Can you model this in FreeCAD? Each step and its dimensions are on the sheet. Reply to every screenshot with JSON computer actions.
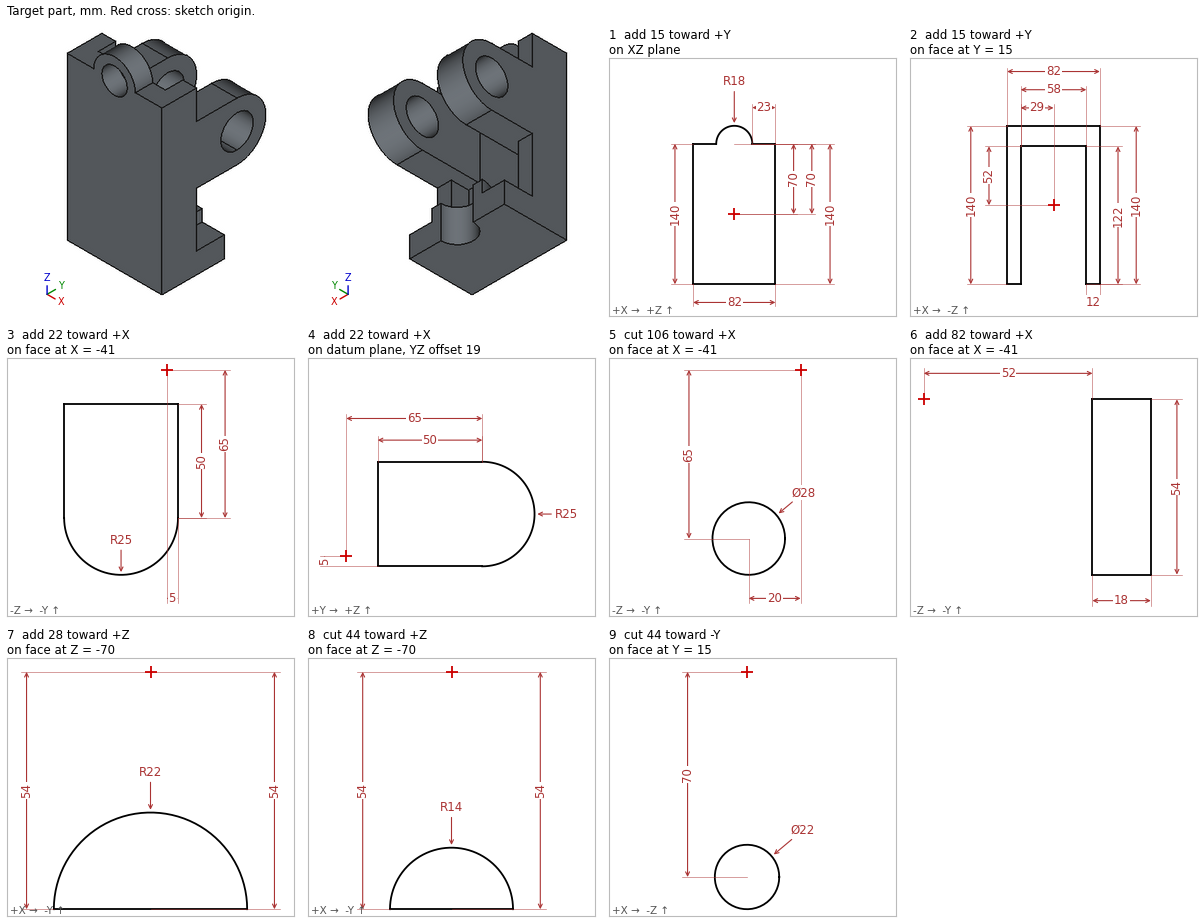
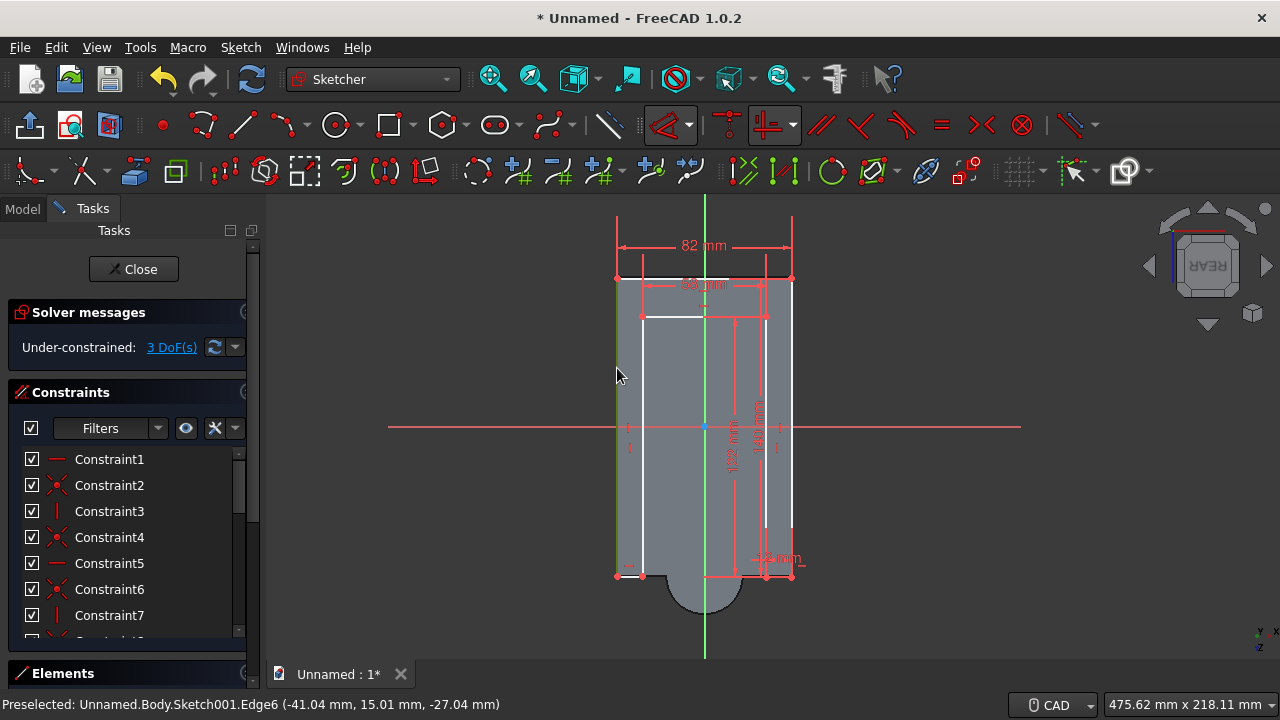
{"action": "key", "text": "i"}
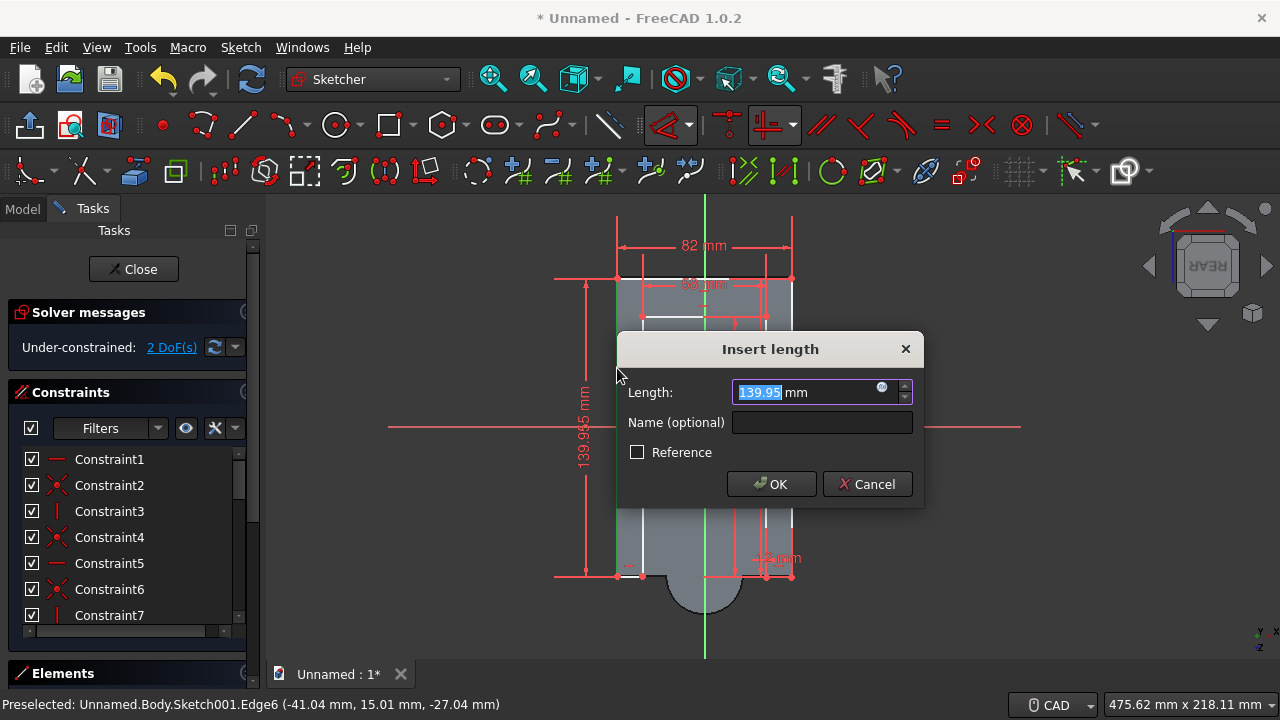
{"action": "type", "text": "140"}
{"action": "key", "text": "Return"}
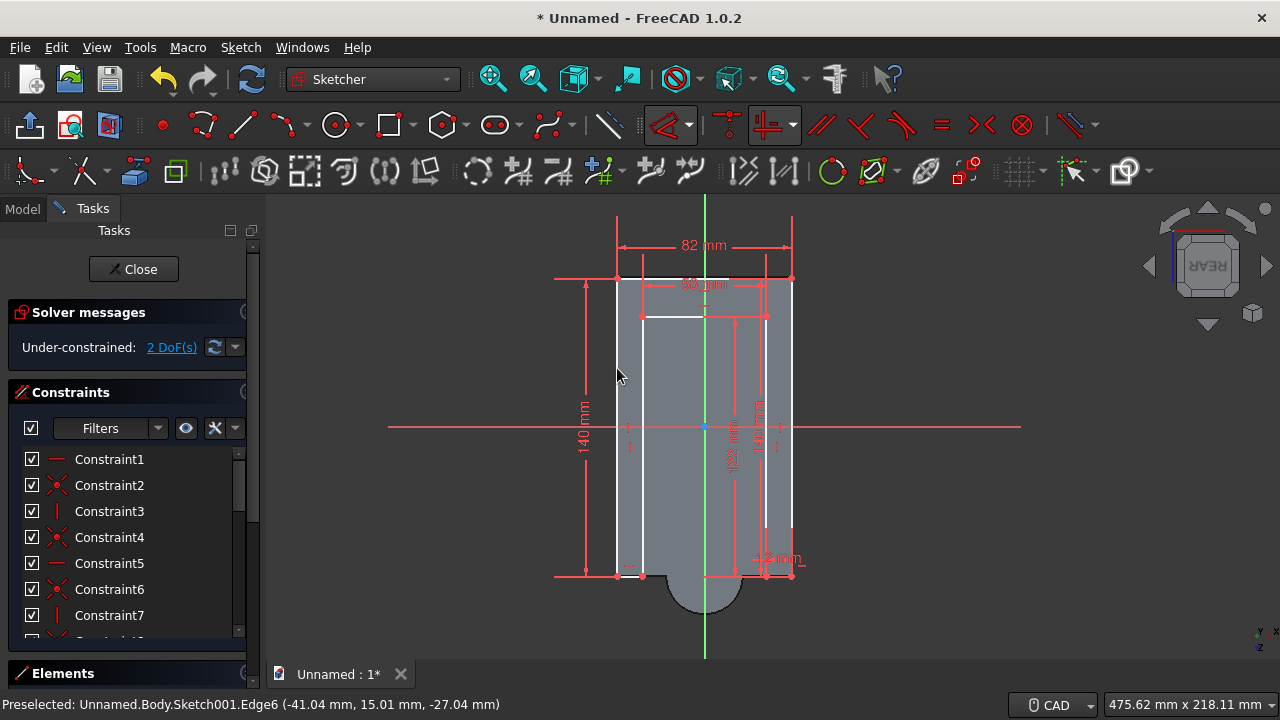
{"action": "left_click", "coordinate": [643, 317]}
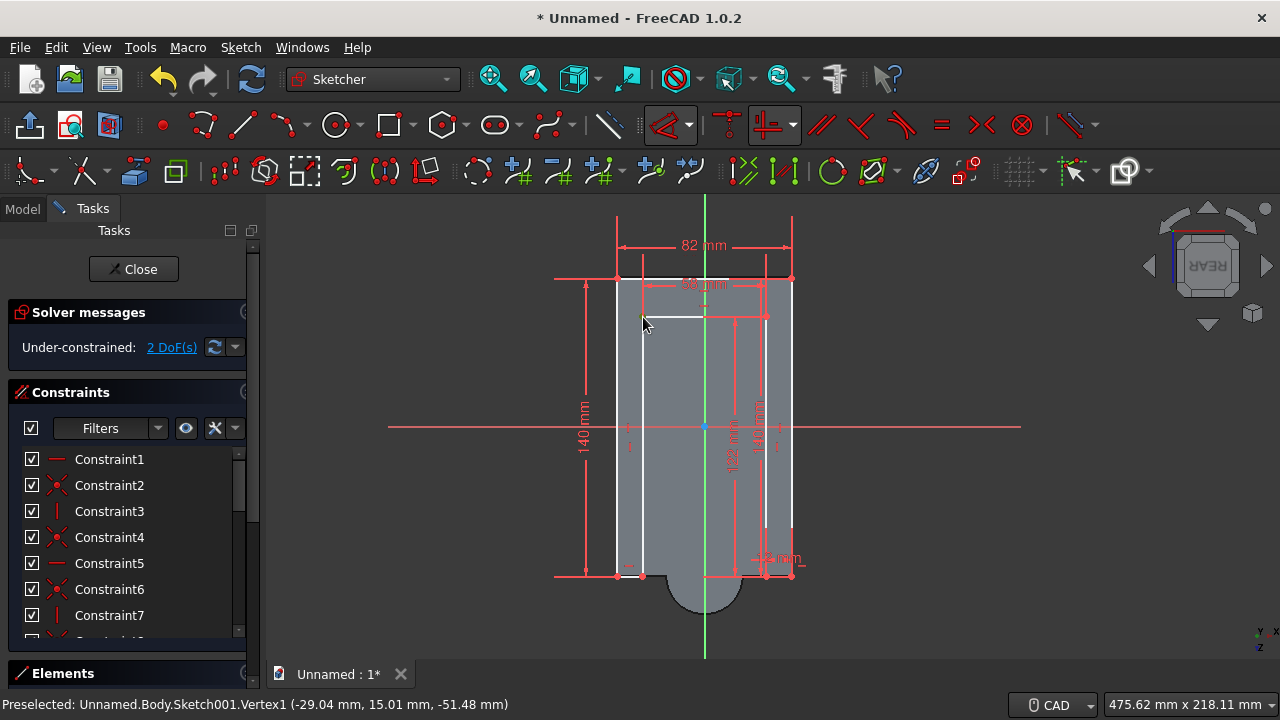
{"action": "key", "text": "l"}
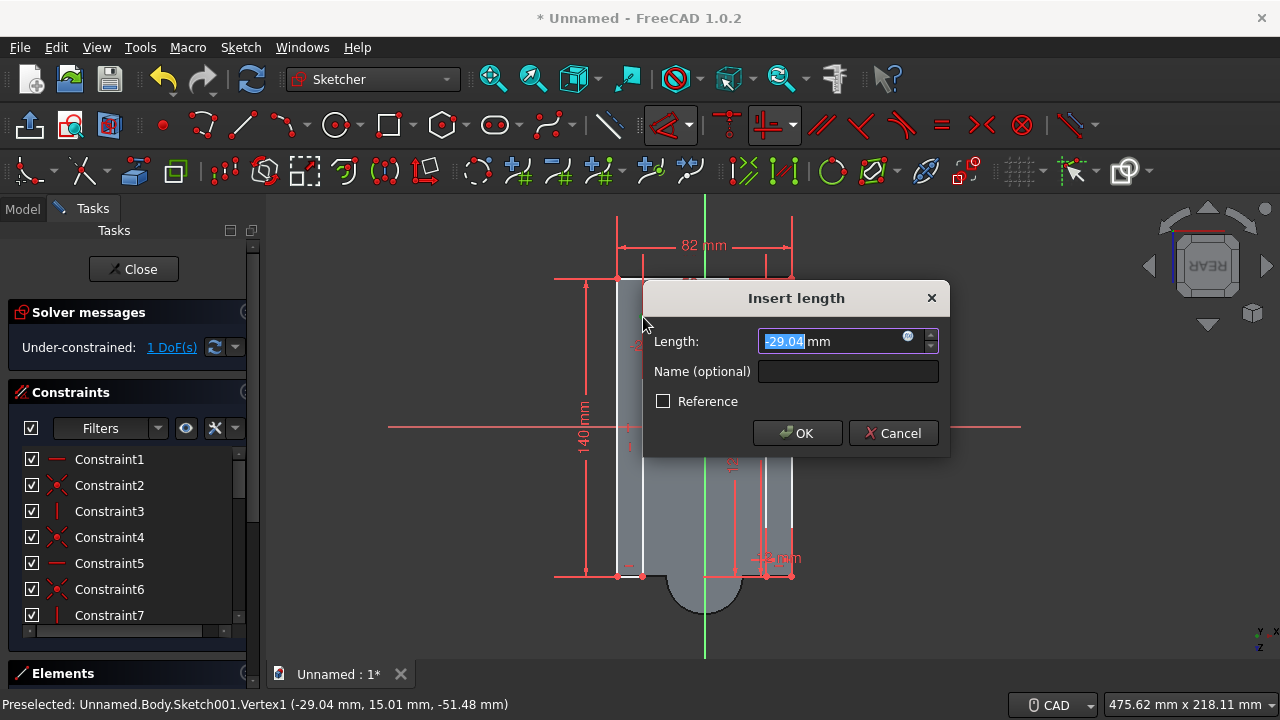
{"action": "type", "text": "-29"}
{"action": "key", "text": "Return"}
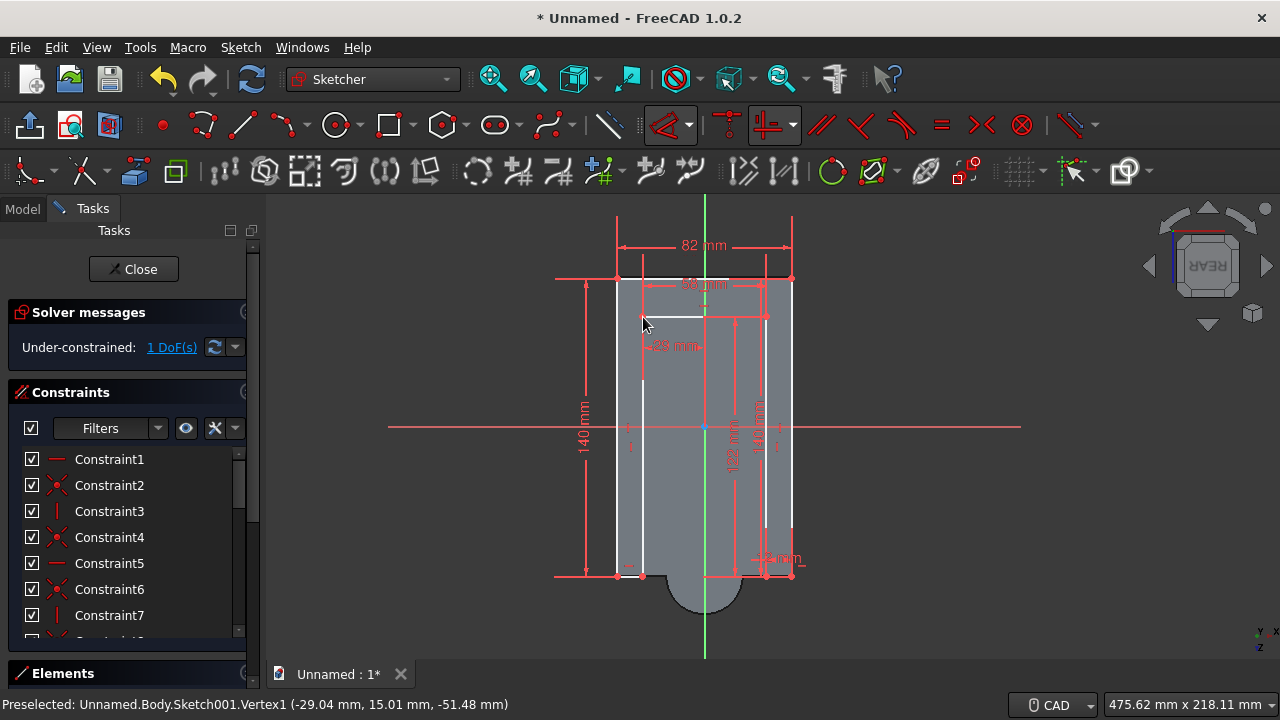
{"action": "left_click", "coordinate": [643, 317]}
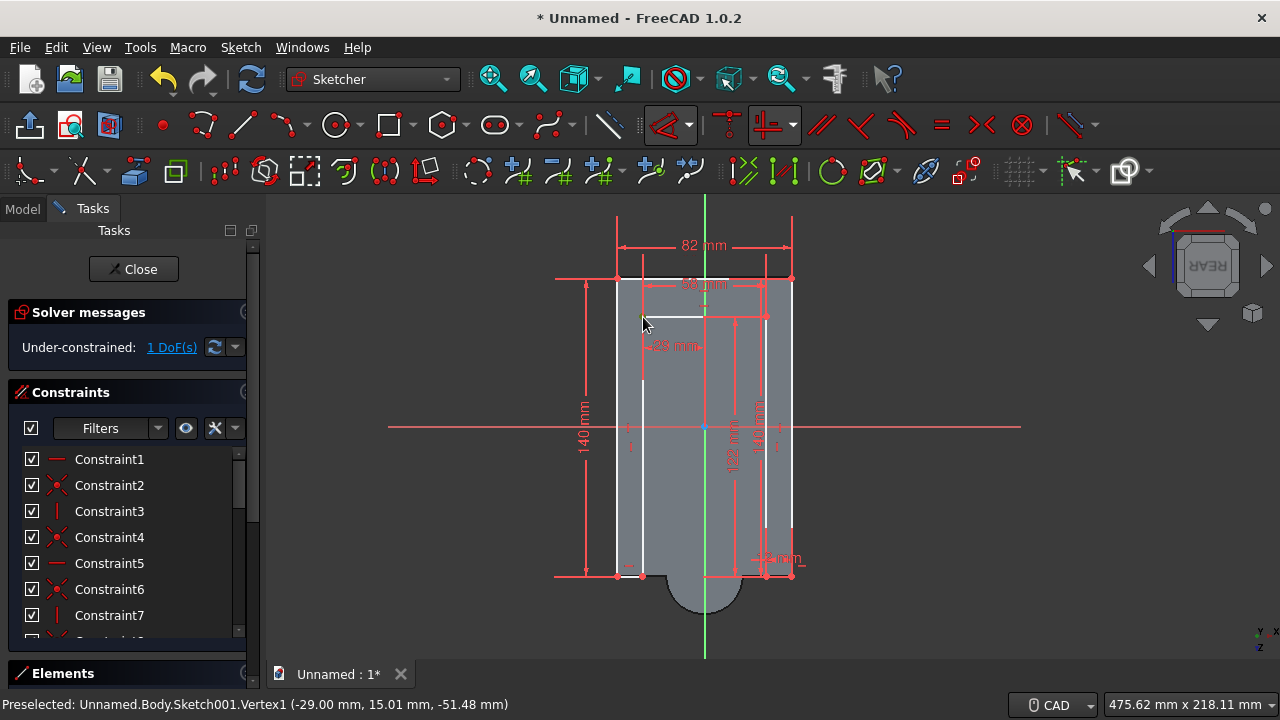
{"action": "key", "text": "i"}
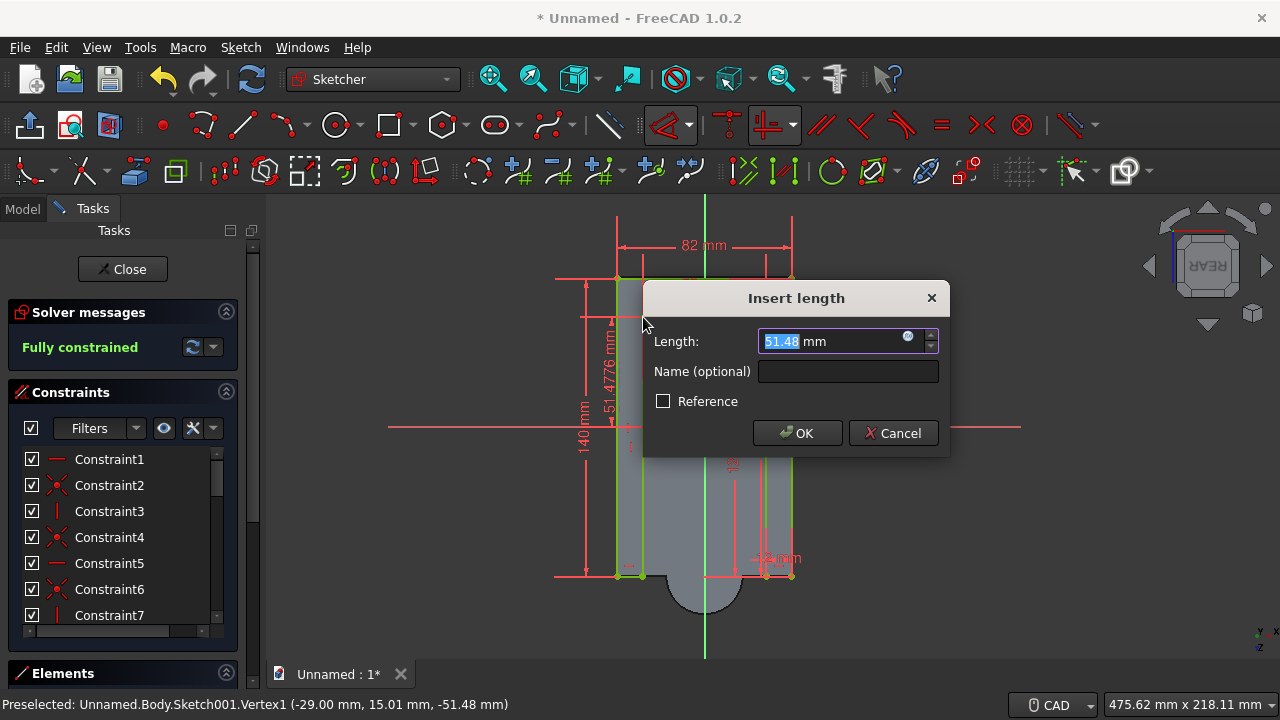
{"action": "type", "text": "52"}
{"action": "key", "text": "Return"}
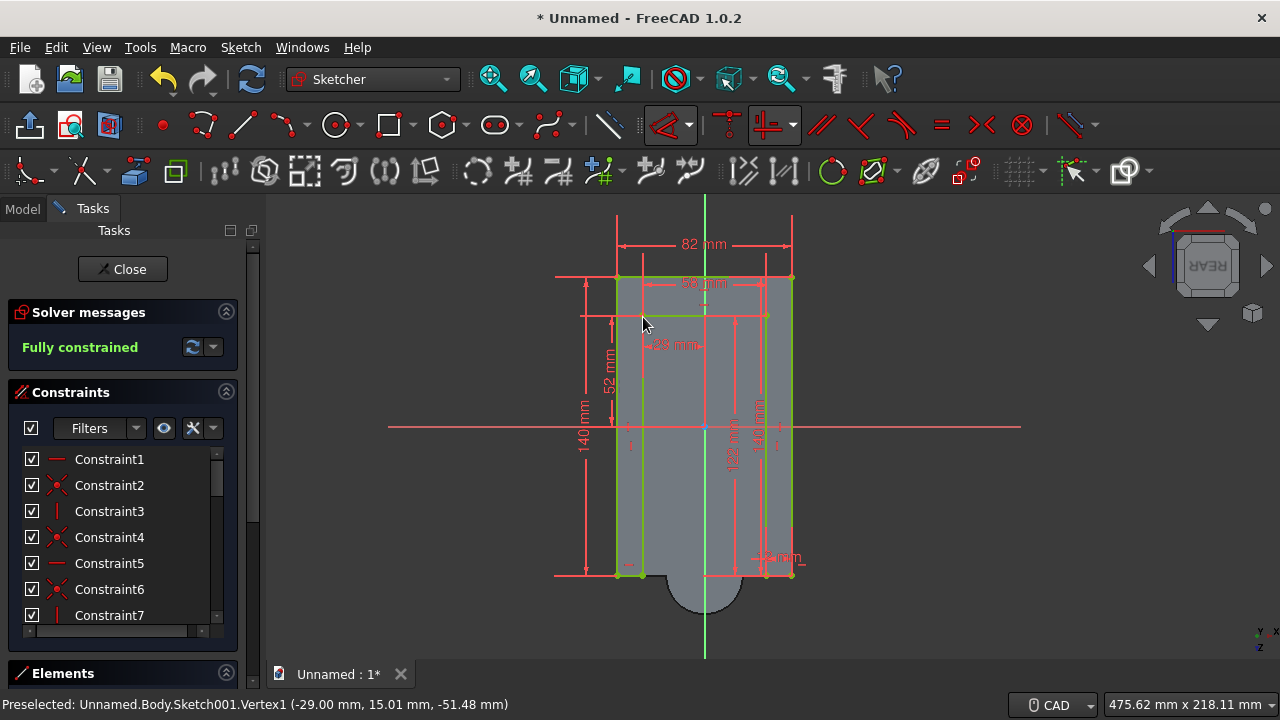
{"action": "left_click", "coordinate": [123, 269]}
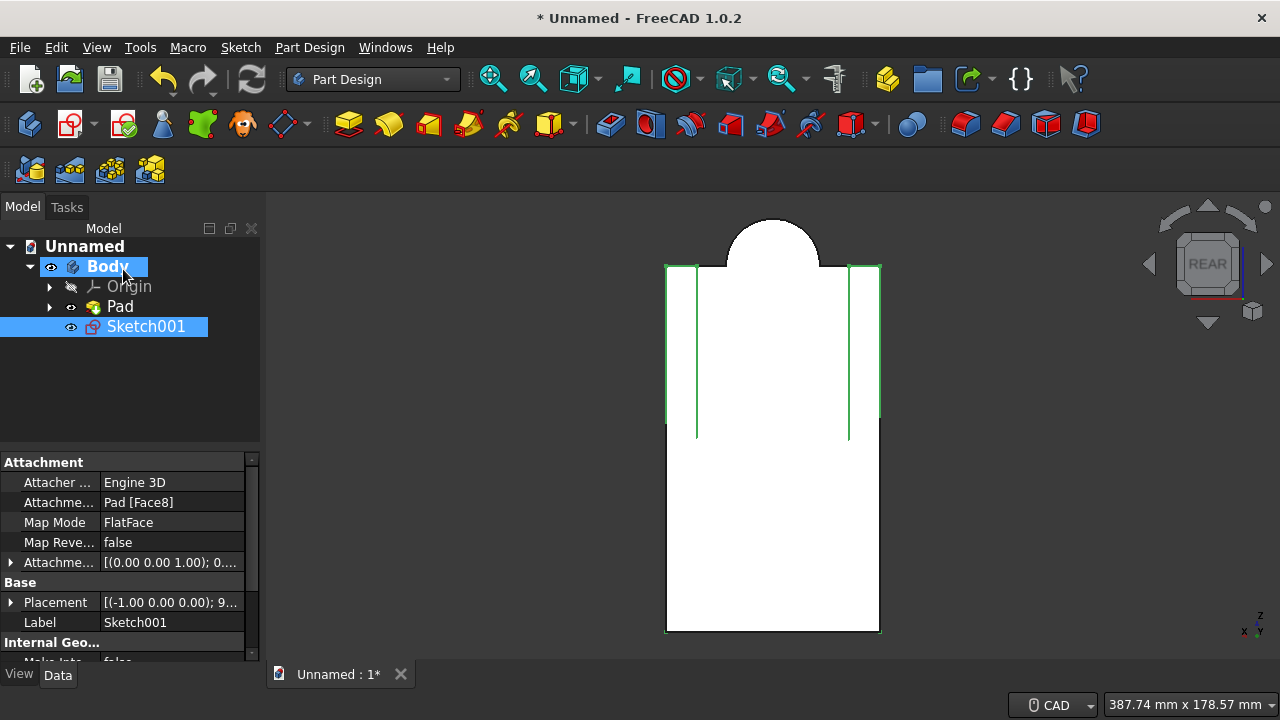
{"action": "left_click", "coordinate": [350, 124]}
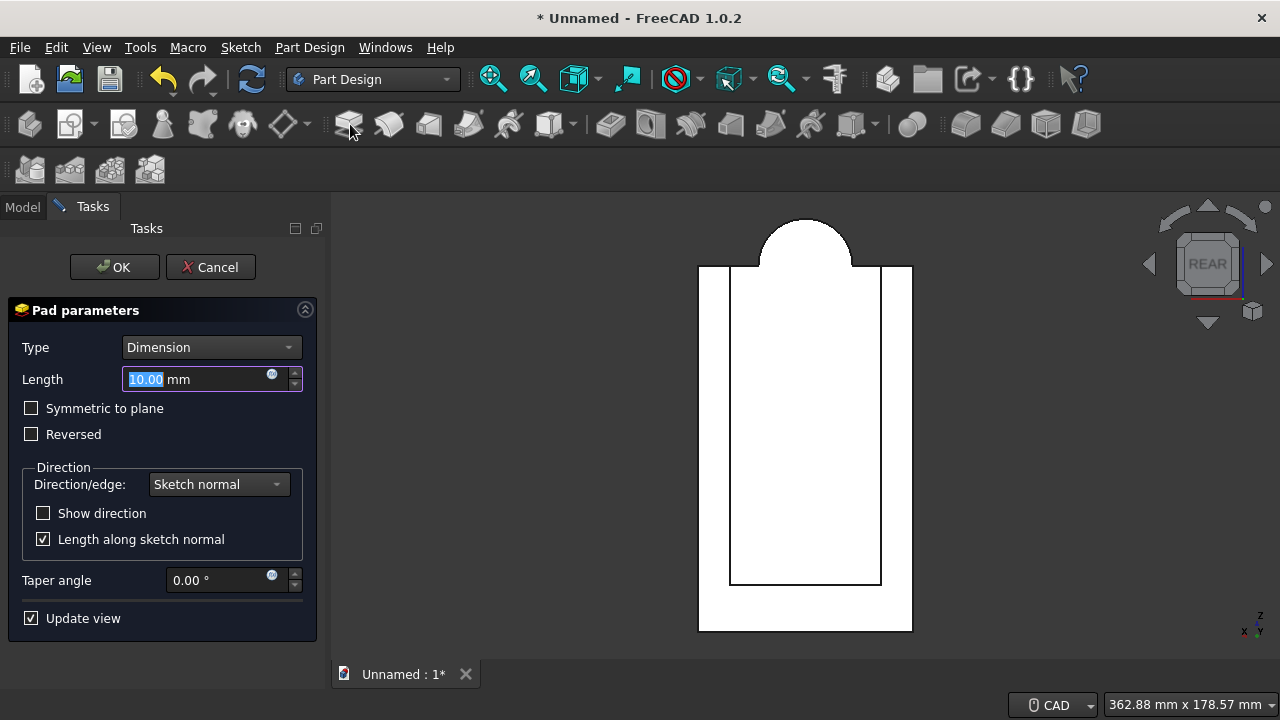
{"action": "type", "text": "15"}
{"action": "key", "text": "Tab"}